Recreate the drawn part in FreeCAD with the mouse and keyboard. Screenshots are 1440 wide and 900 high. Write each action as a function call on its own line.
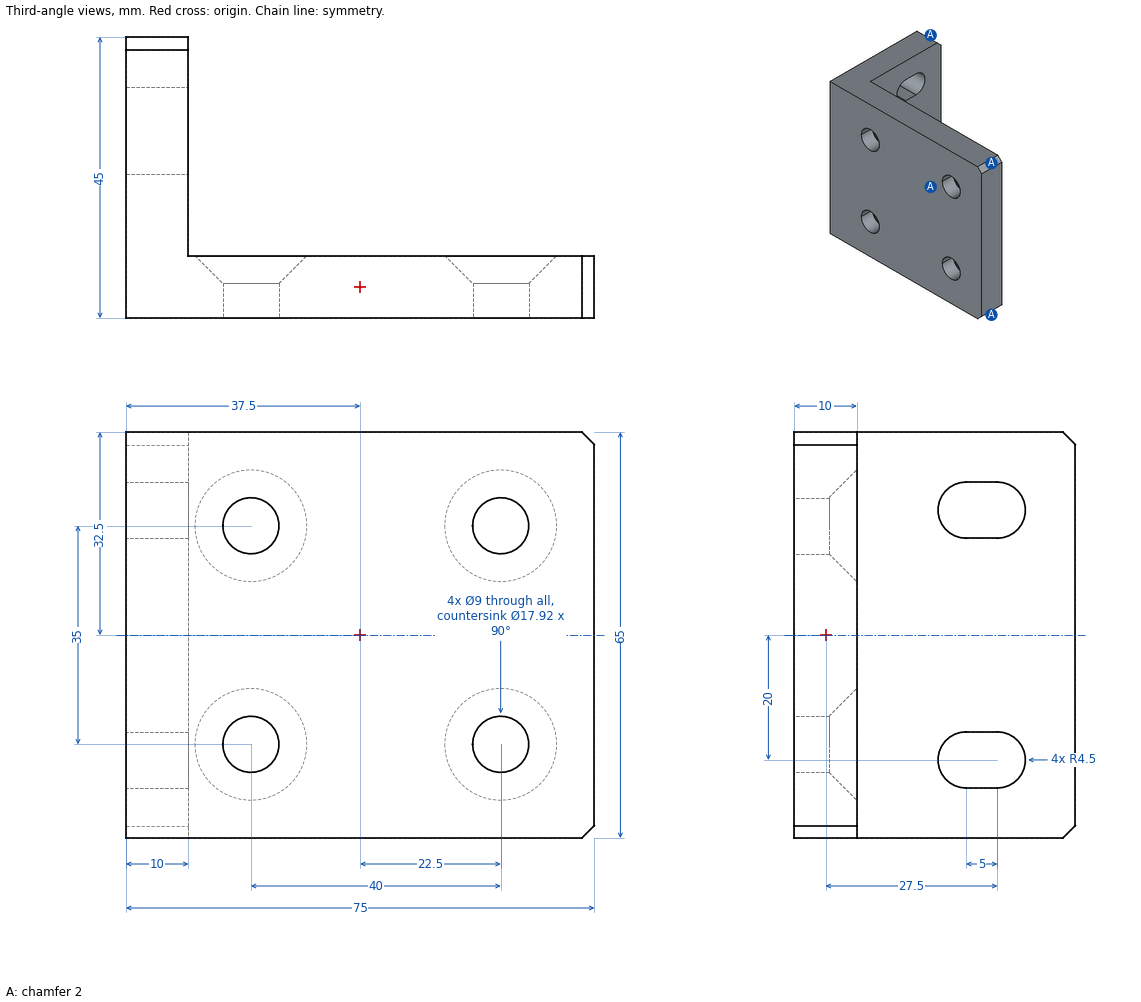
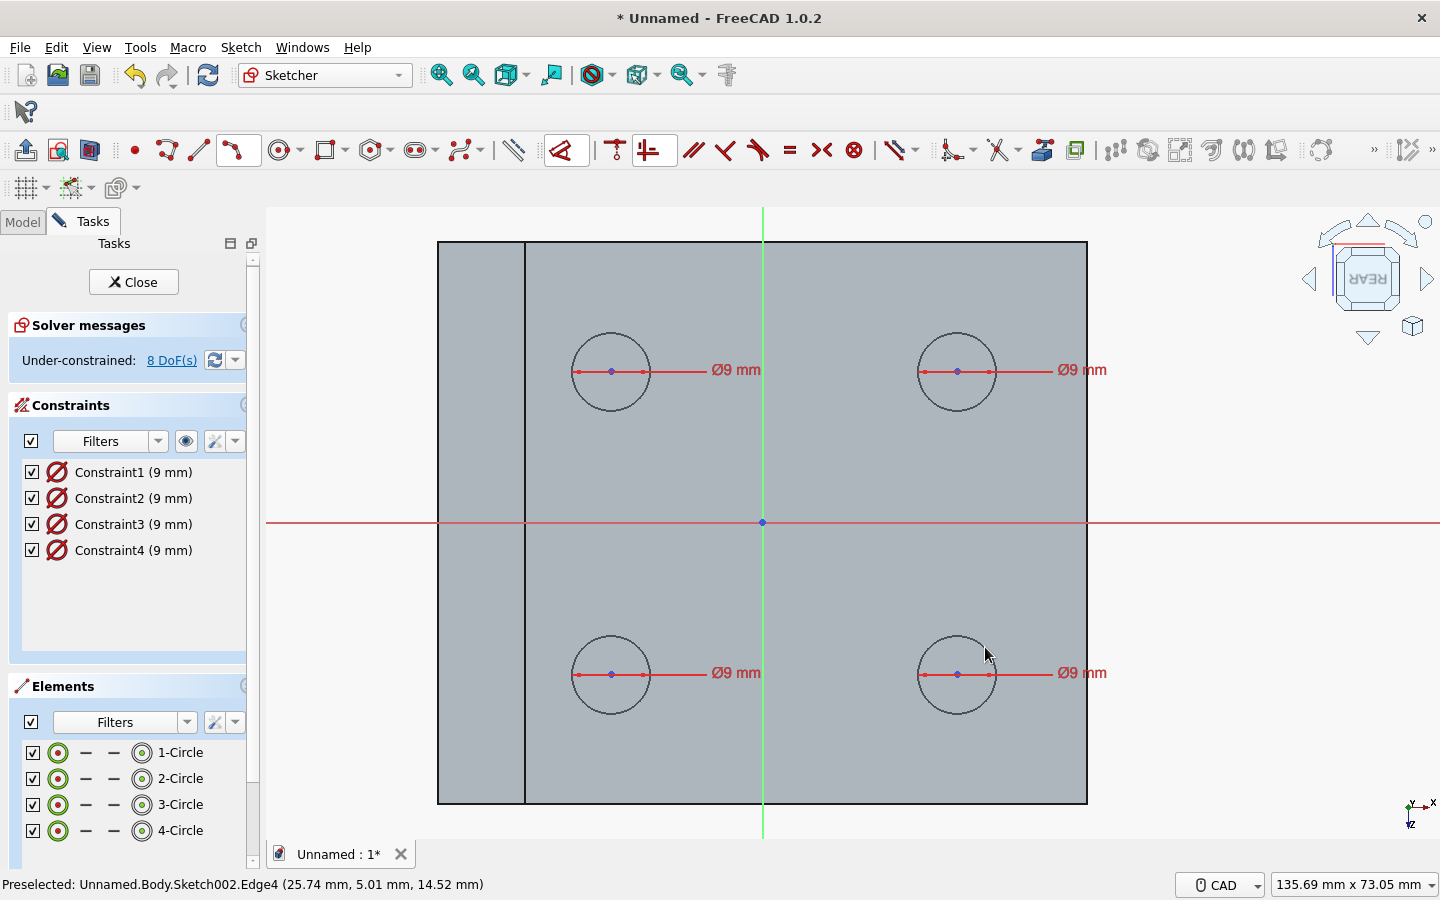
click(611, 372)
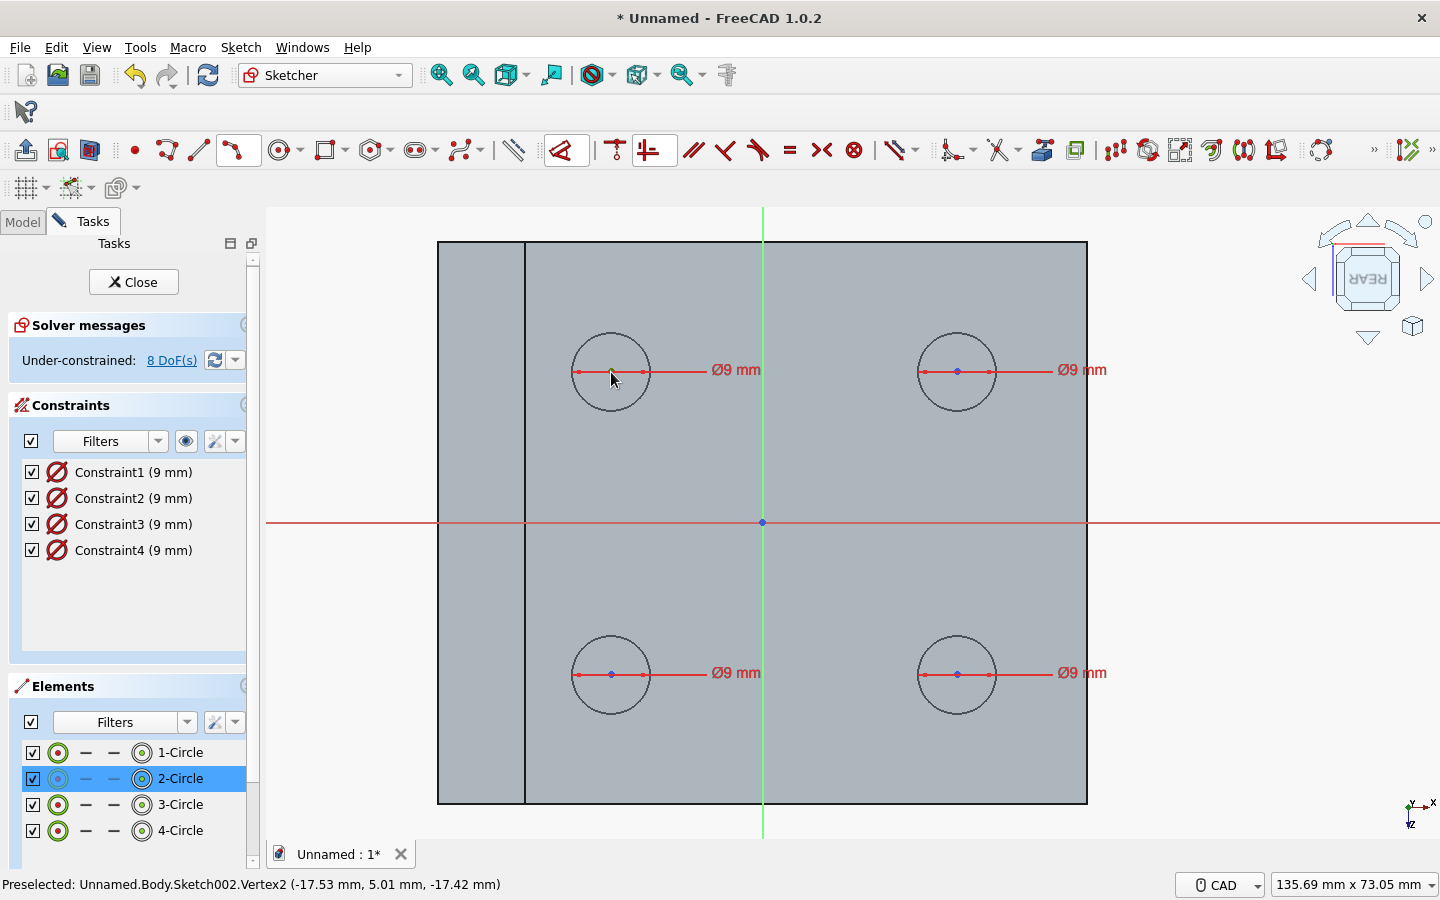
click(611, 675)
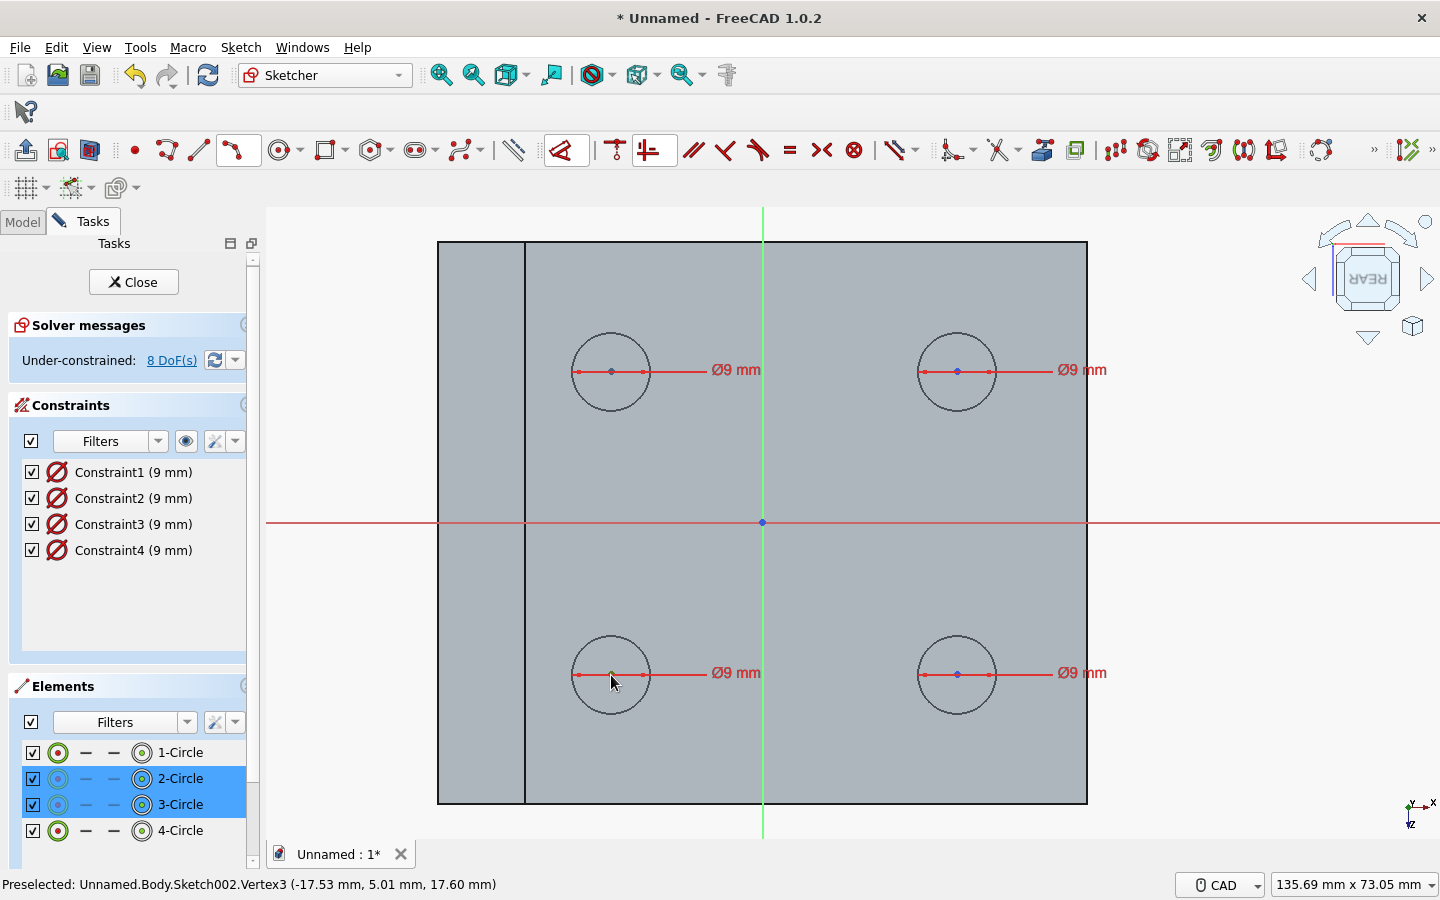
click(364, 523)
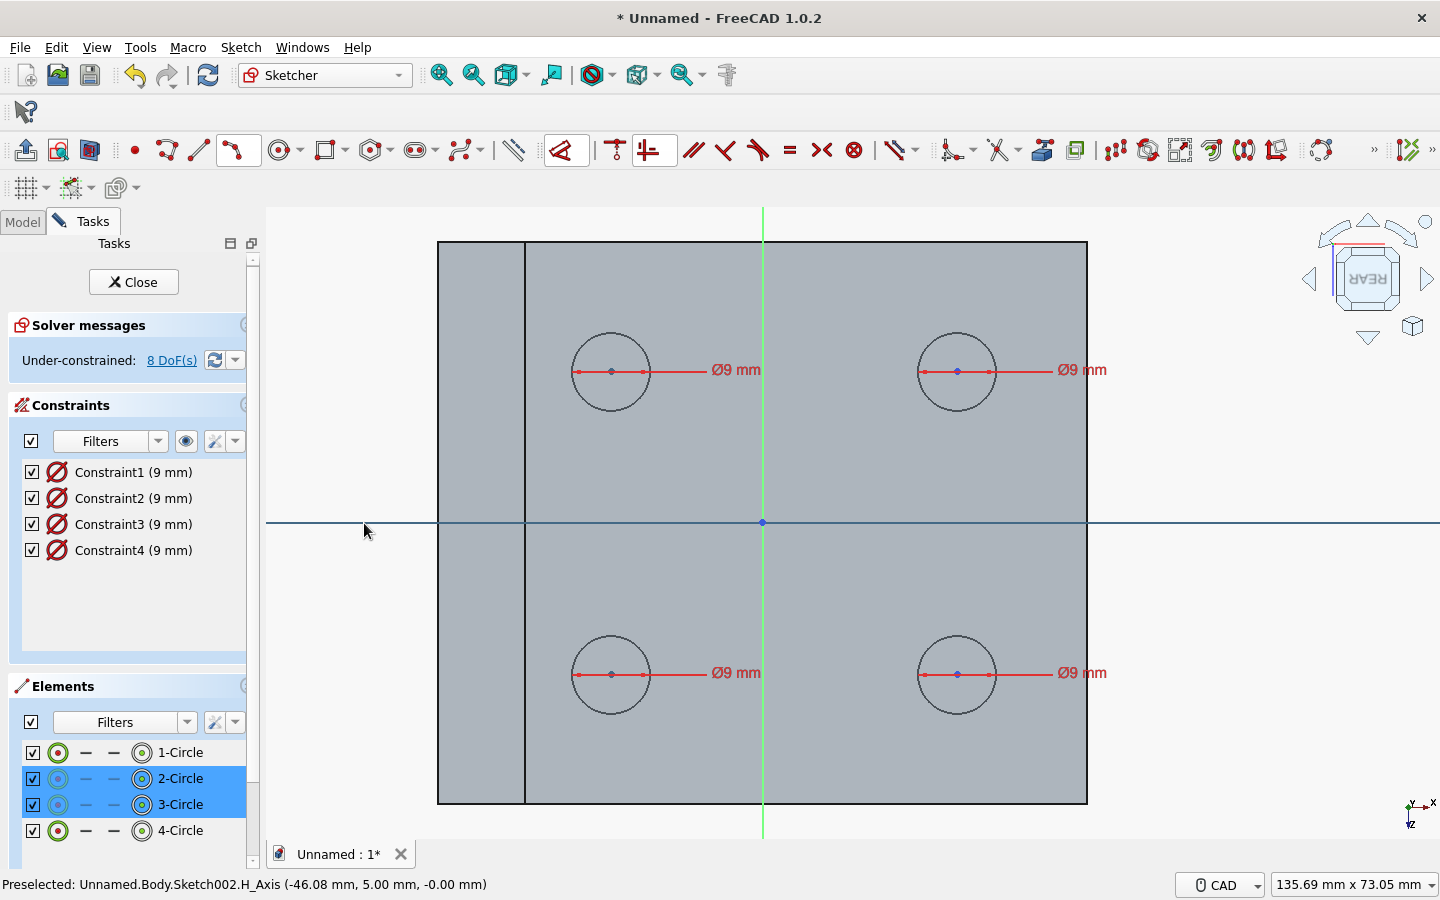
key(s)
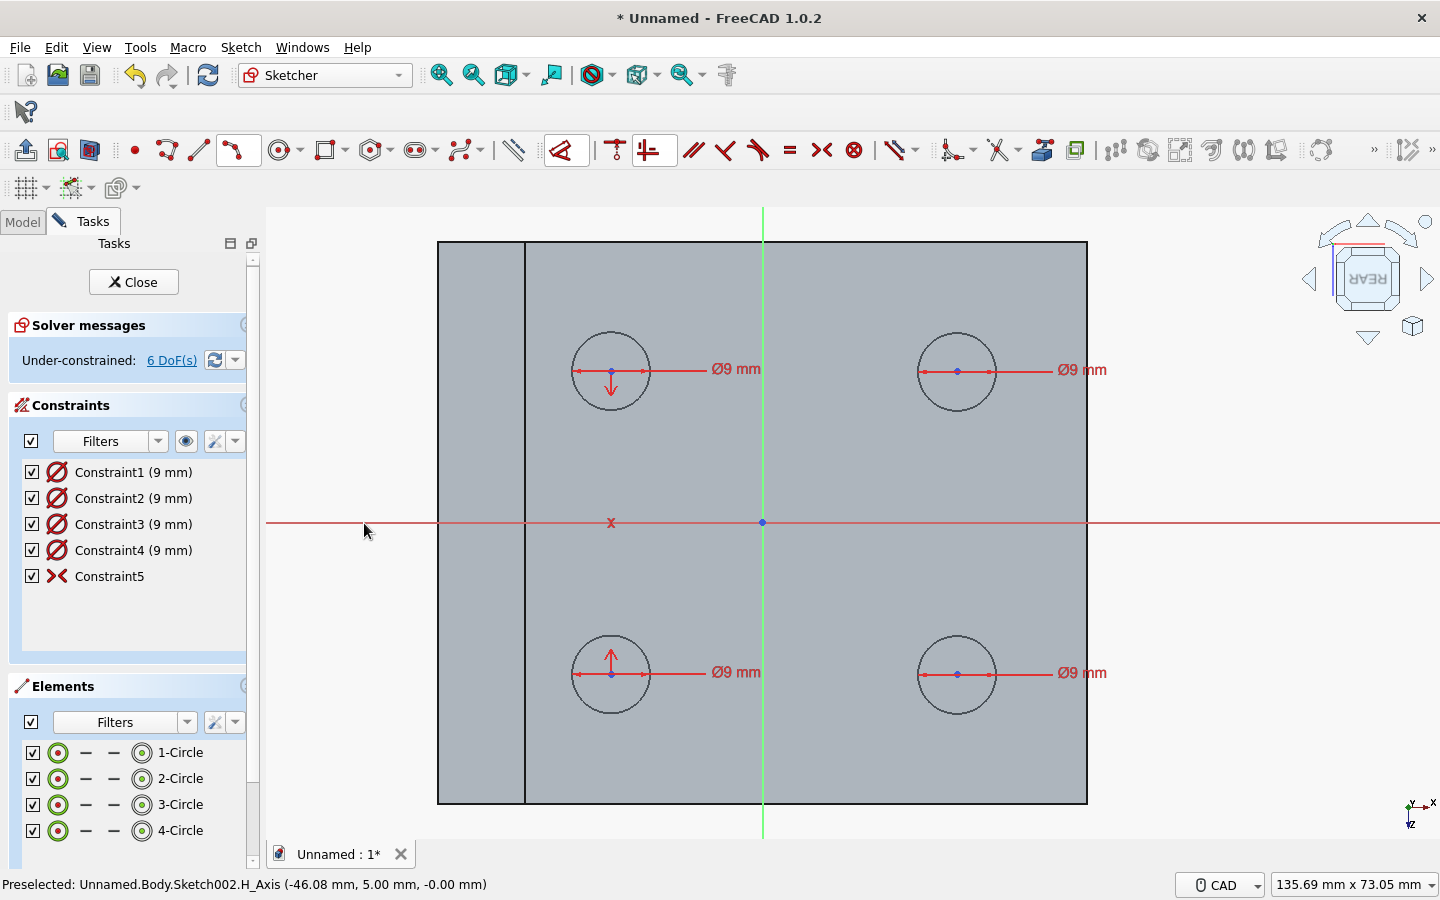
click(957, 372)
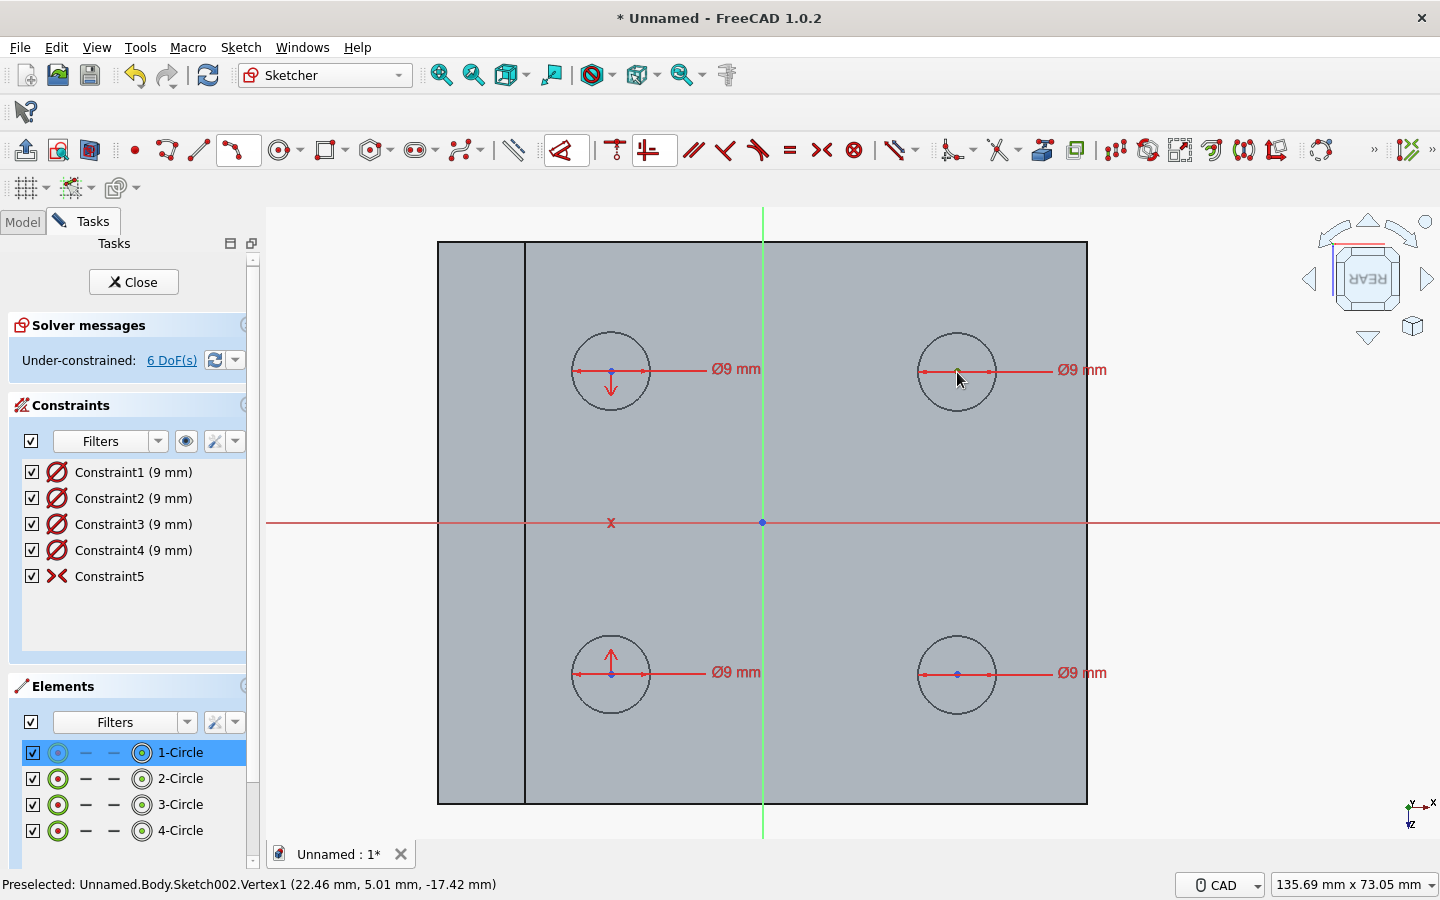
click(957, 675)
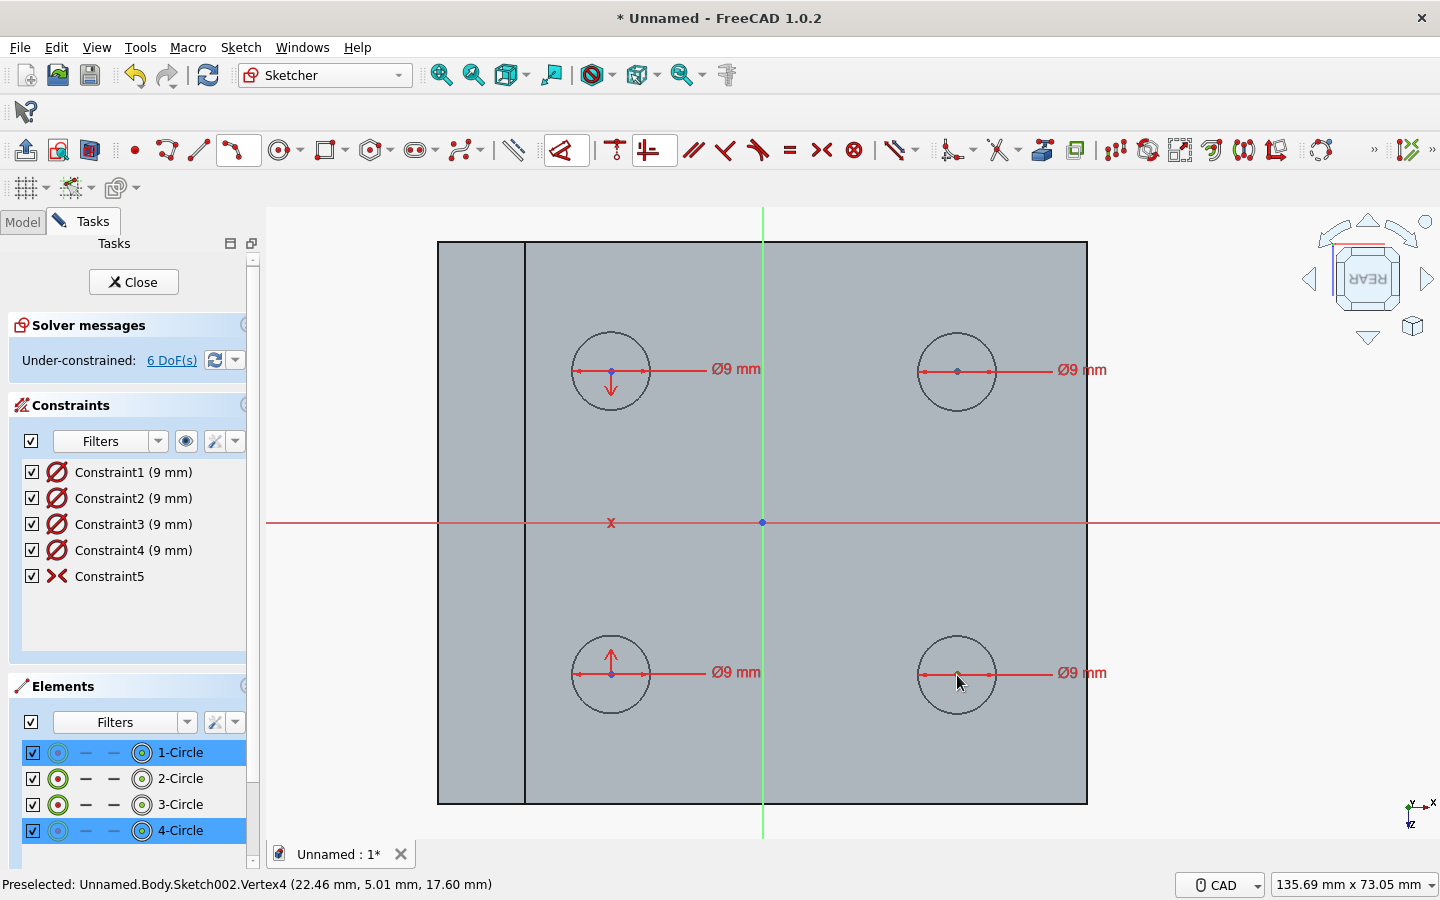
click(364, 523)